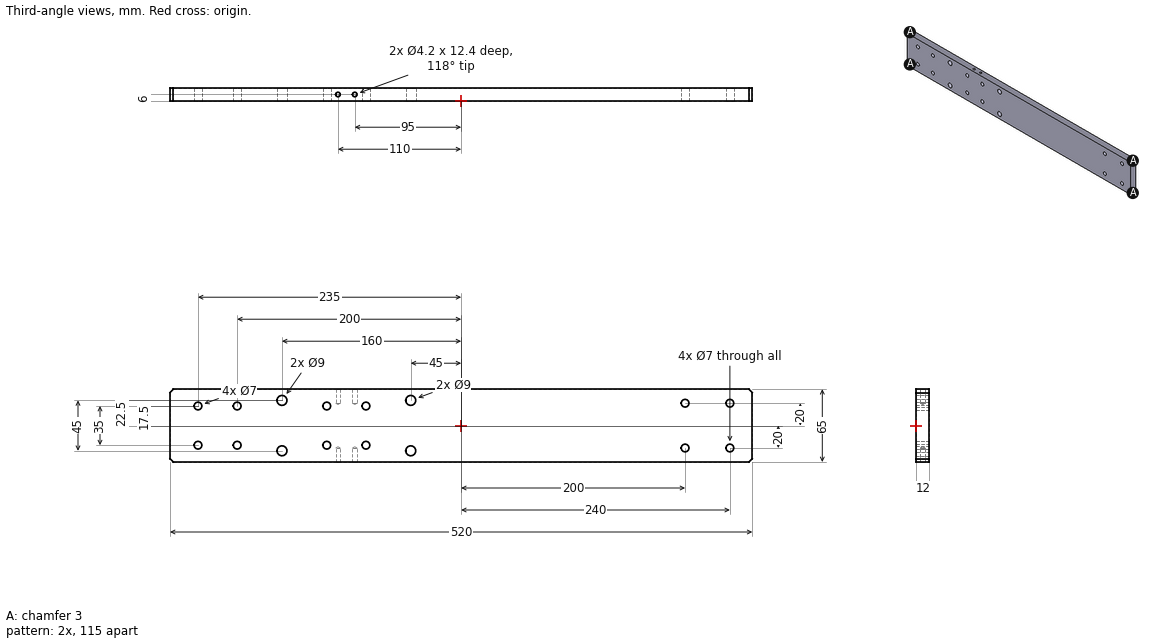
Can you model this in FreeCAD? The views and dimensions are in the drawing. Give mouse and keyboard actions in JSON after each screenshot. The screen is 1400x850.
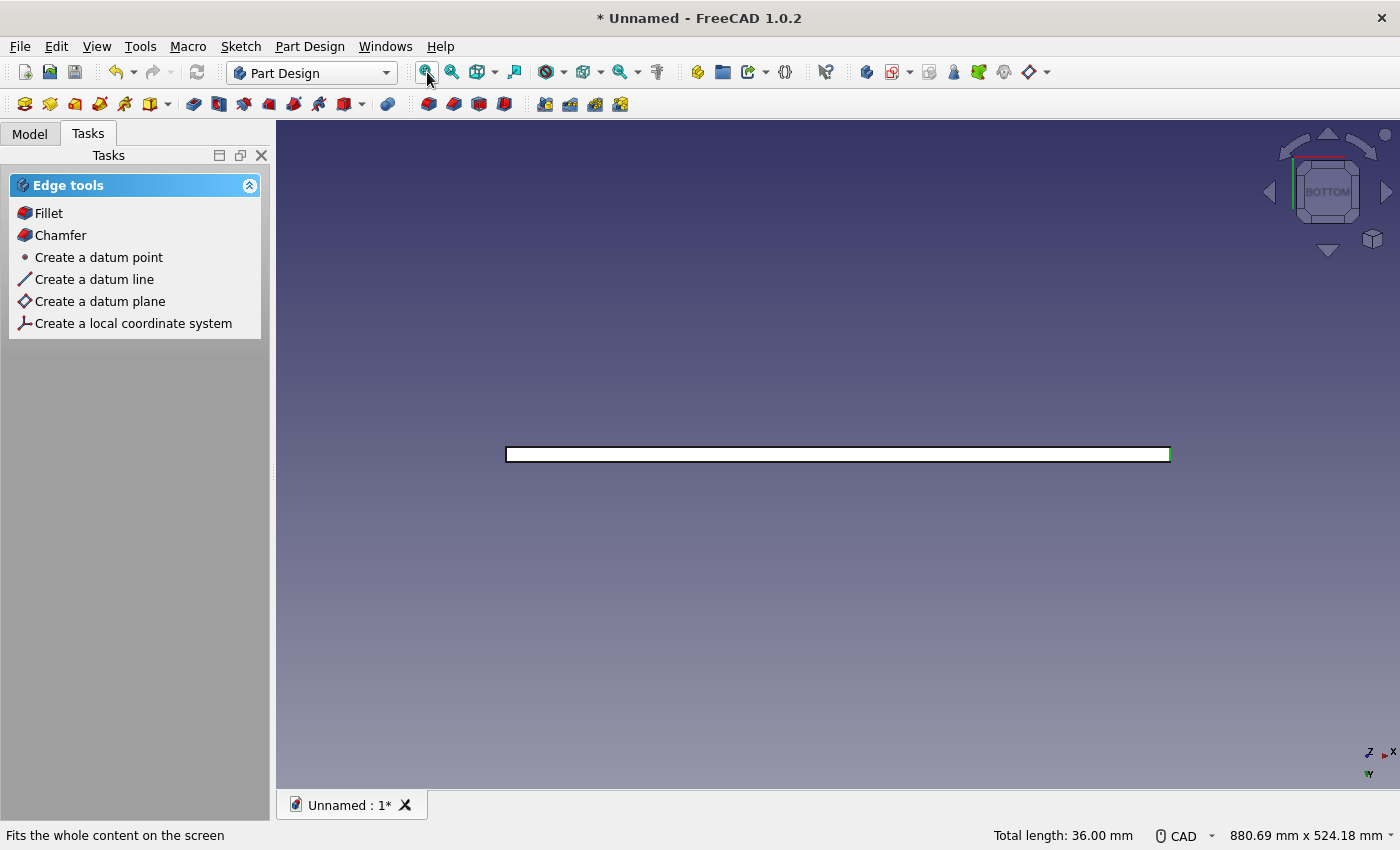
{"action": "left_click", "coordinate": [506, 453], "text": "ctrl"}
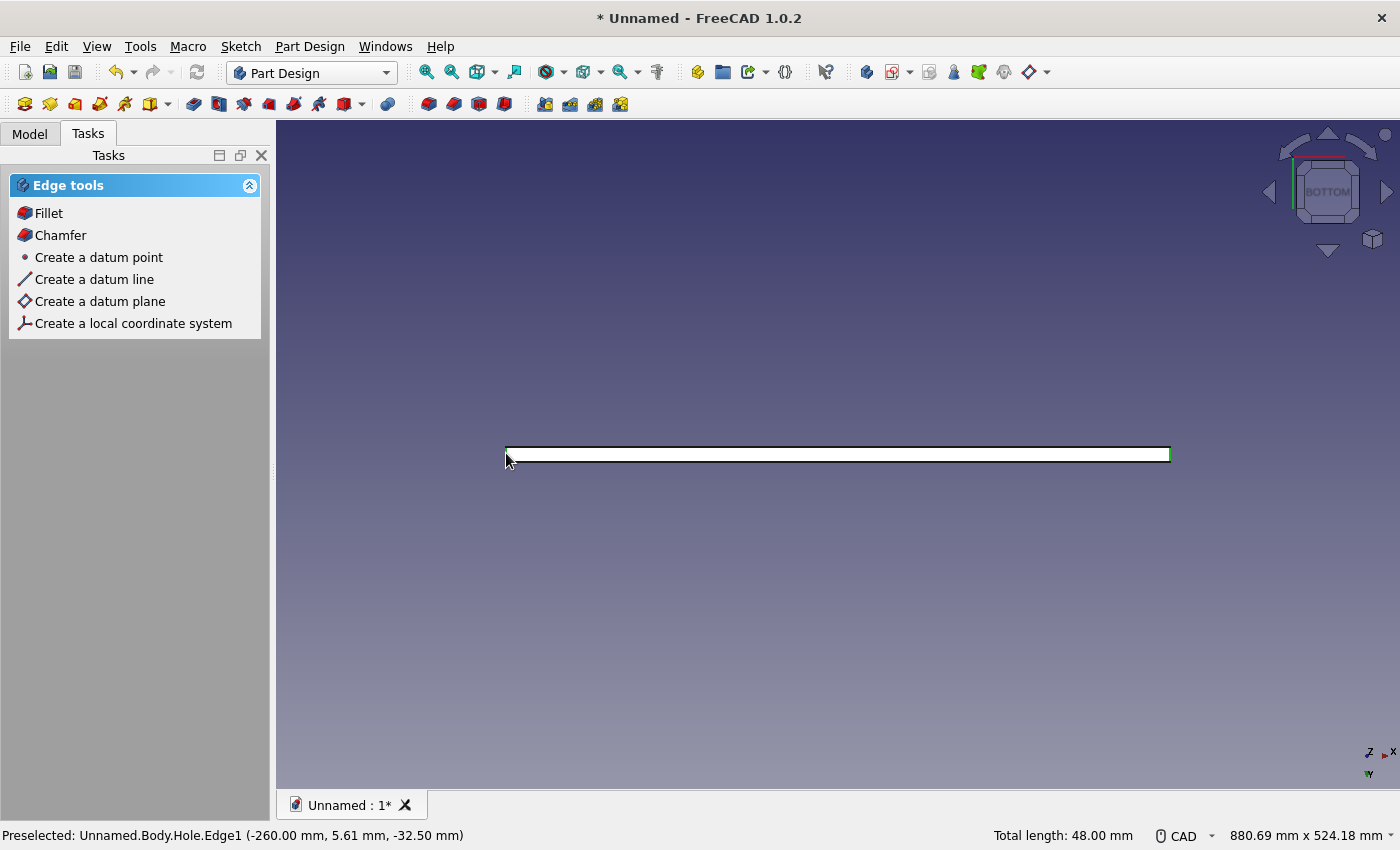
{"action": "left_click", "coordinate": [454, 104]}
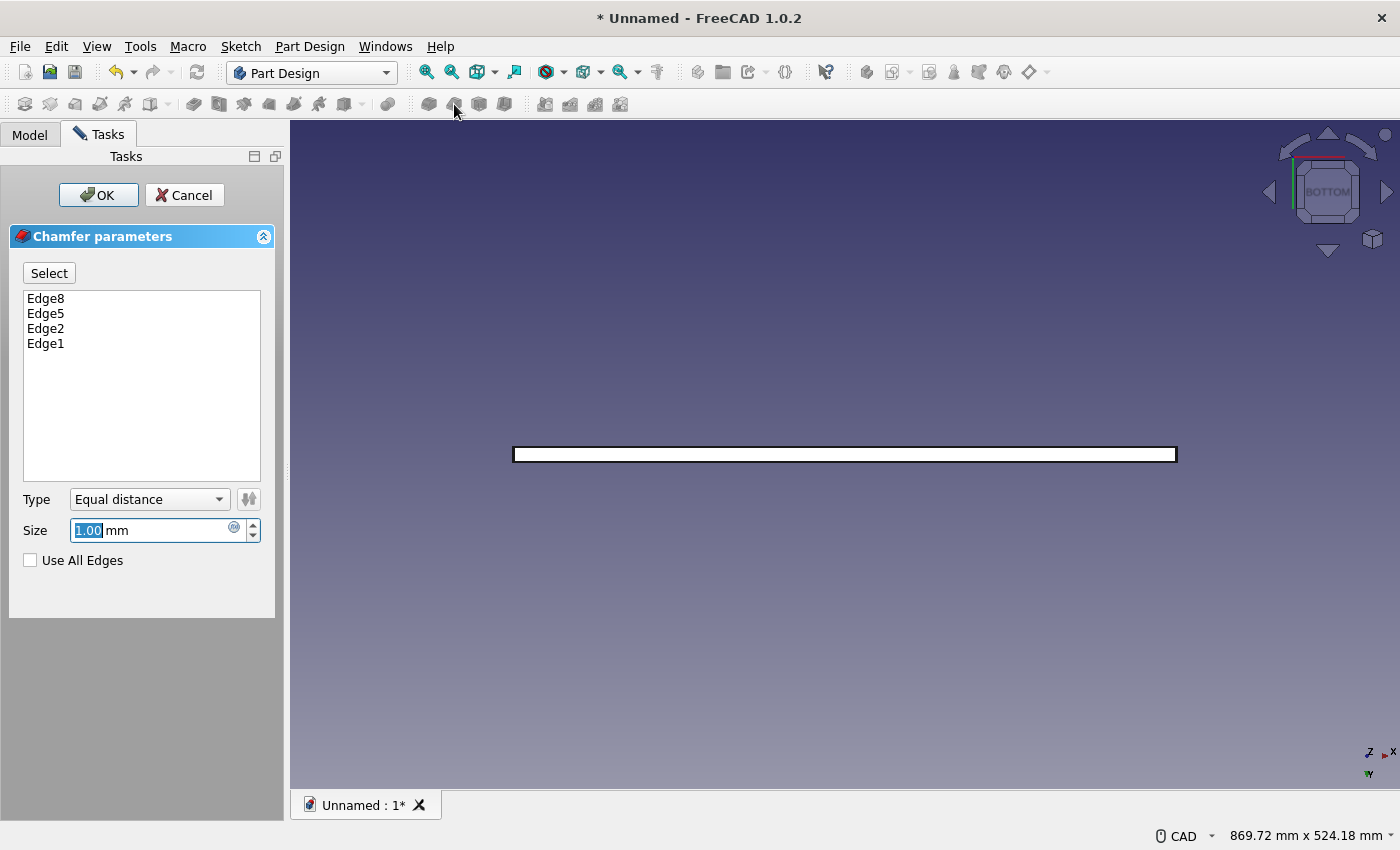
{"action": "type", "text": "3"}
{"action": "key", "text": "Tab"}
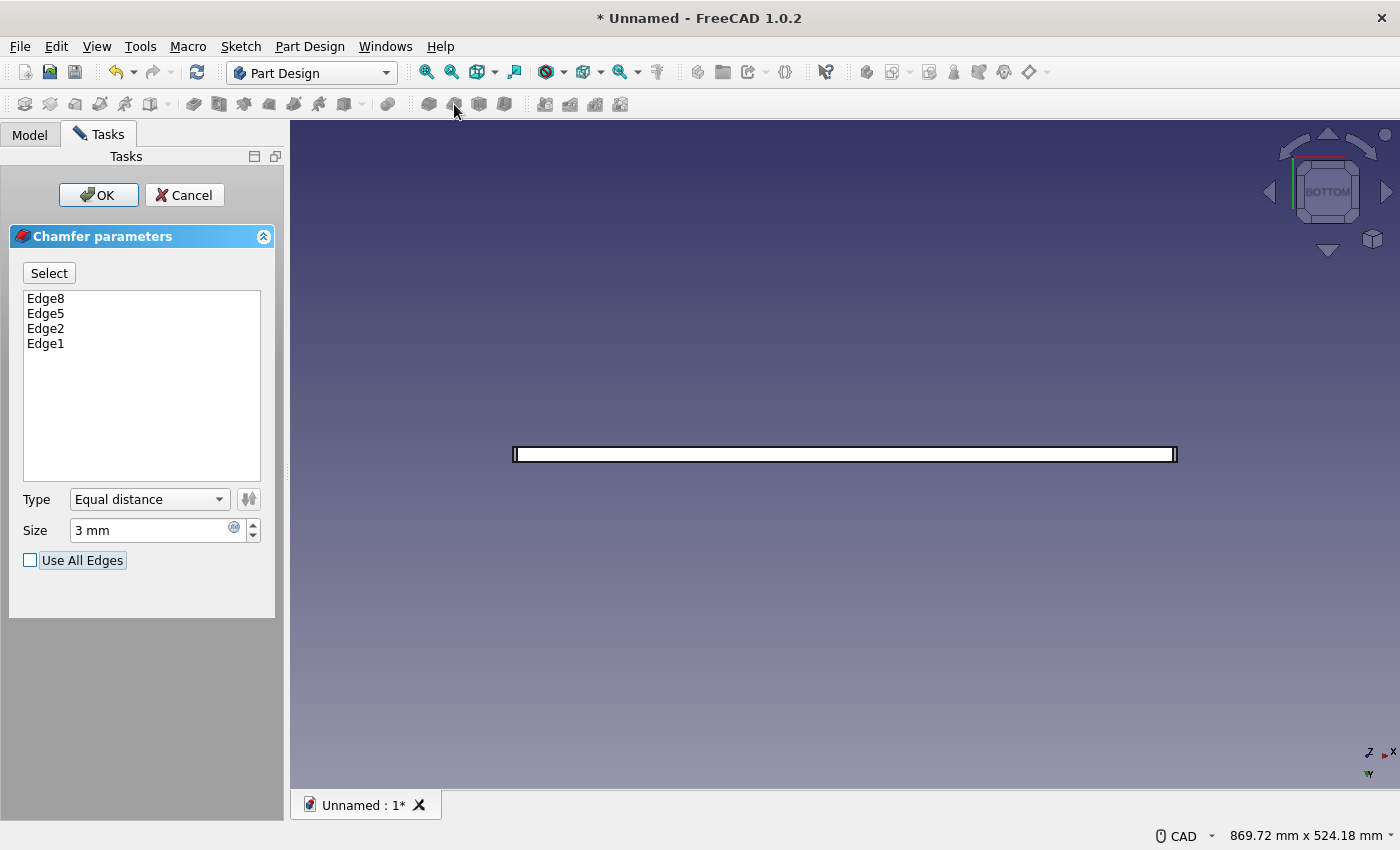
{"action": "left_click", "coordinate": [99, 195]}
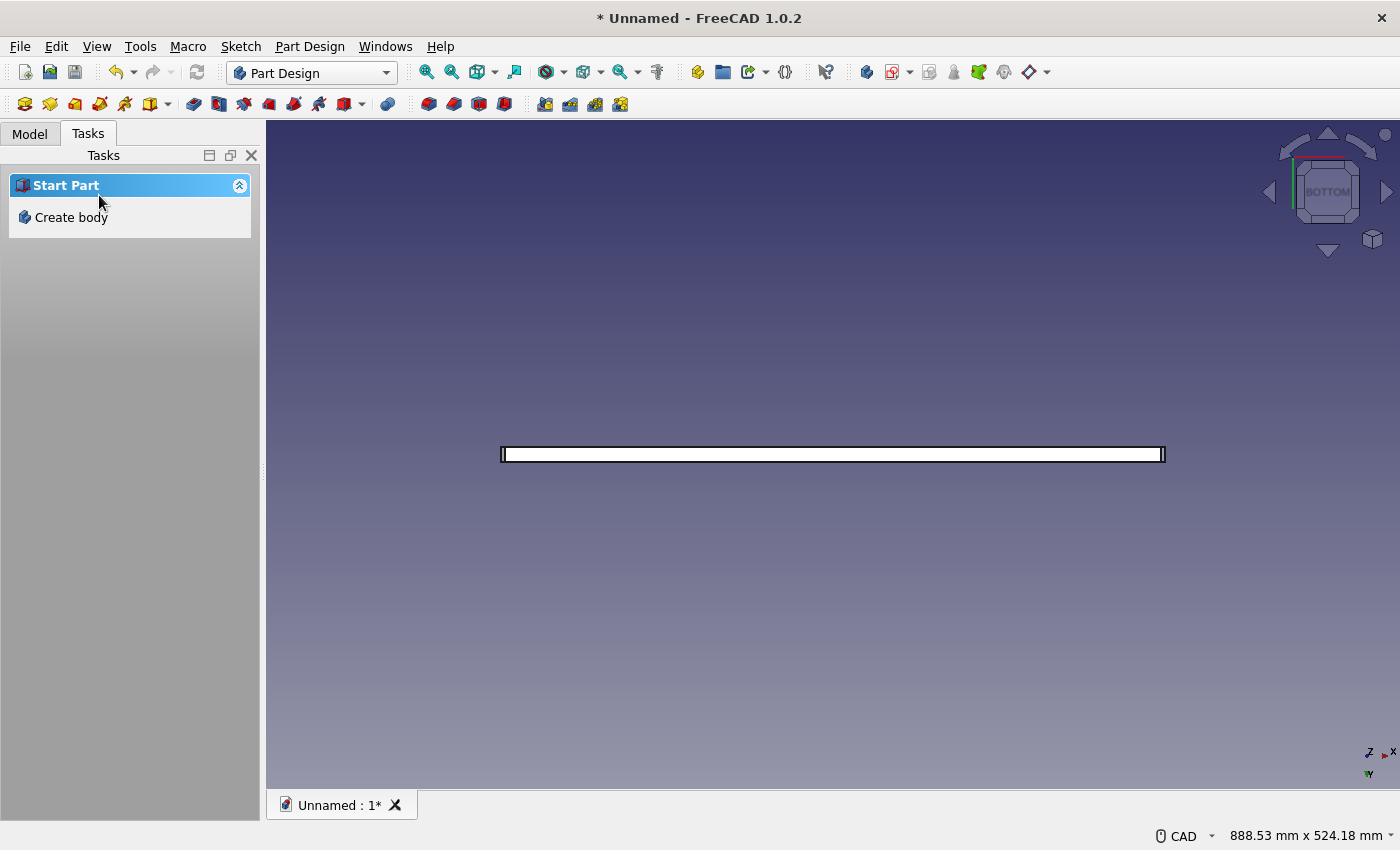
{"action": "key", "text": "4"}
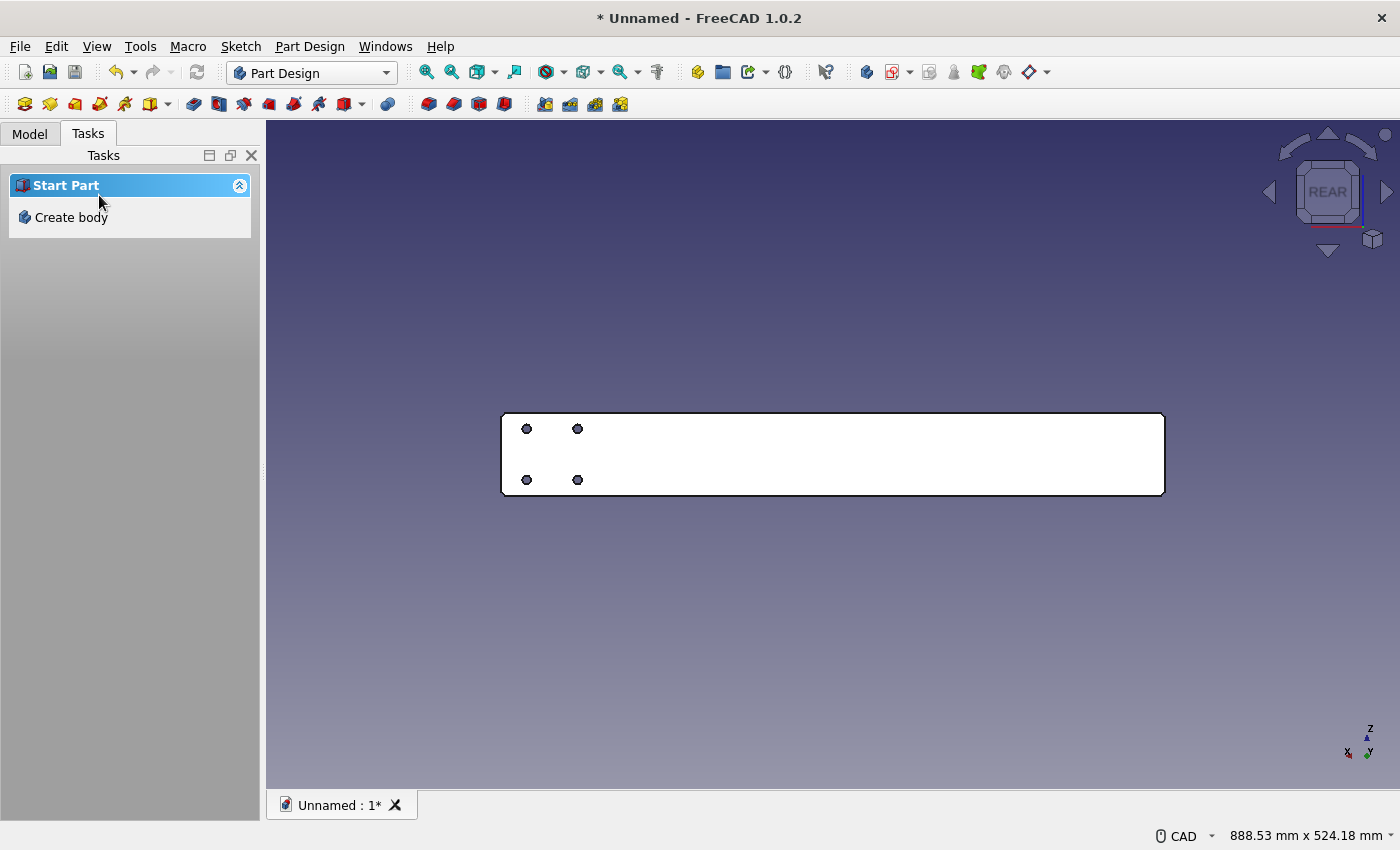
{"action": "left_click", "coordinate": [643, 454]}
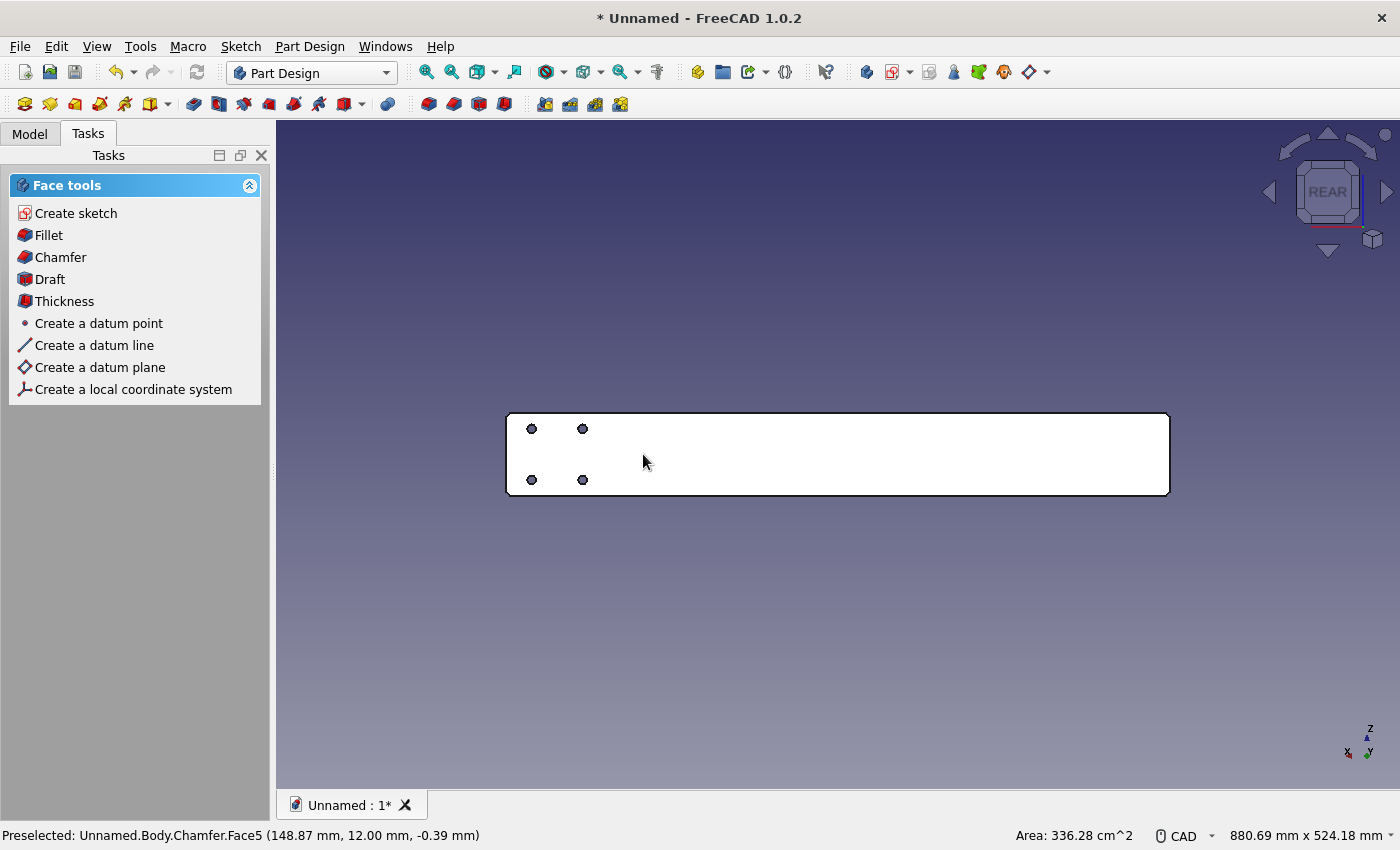
{"action": "left_click", "coordinate": [892, 72]}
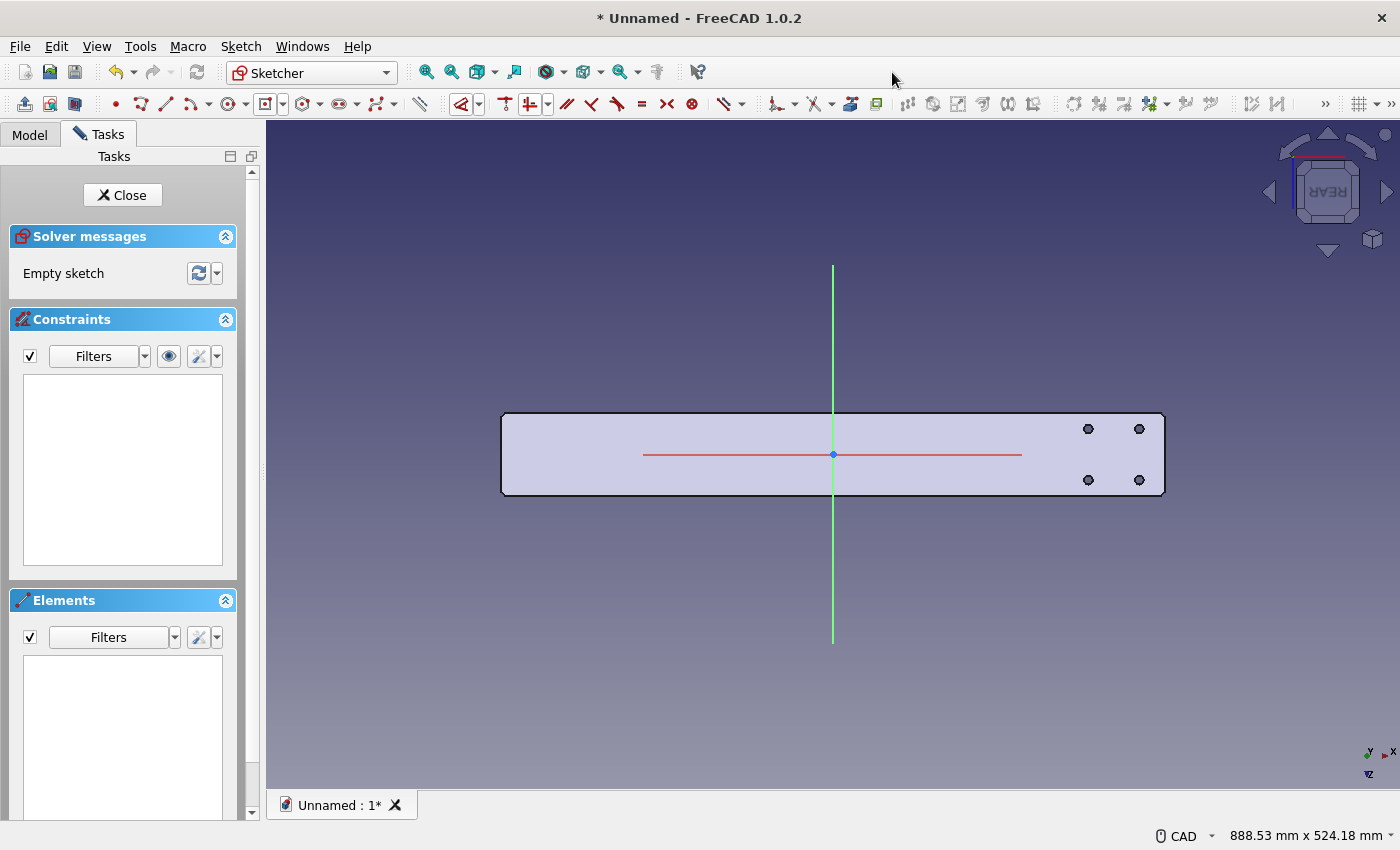
{"action": "scroll", "coordinate": [602, 454], "scroll_direction": "up", "scroll_amount": 9}